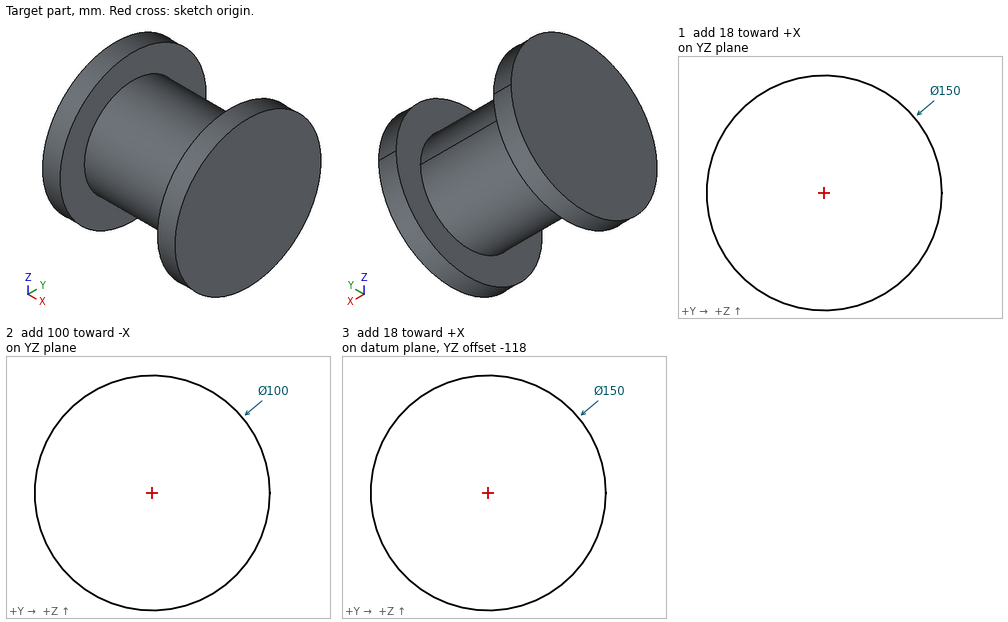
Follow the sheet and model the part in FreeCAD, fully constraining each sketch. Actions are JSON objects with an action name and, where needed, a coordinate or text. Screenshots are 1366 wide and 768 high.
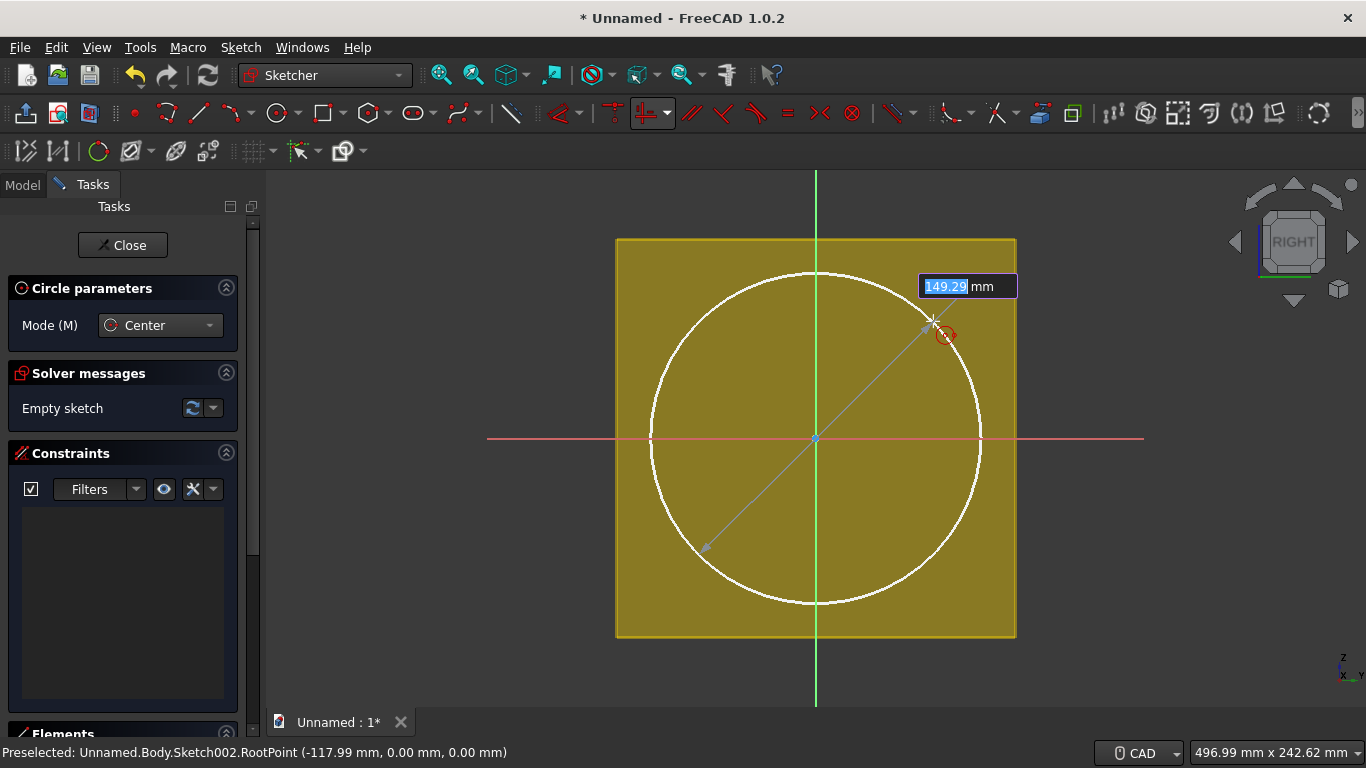
{"action": "type", "text": "150"}
{"action": "key", "text": "Return"}
{"action": "key", "text": "Escape"}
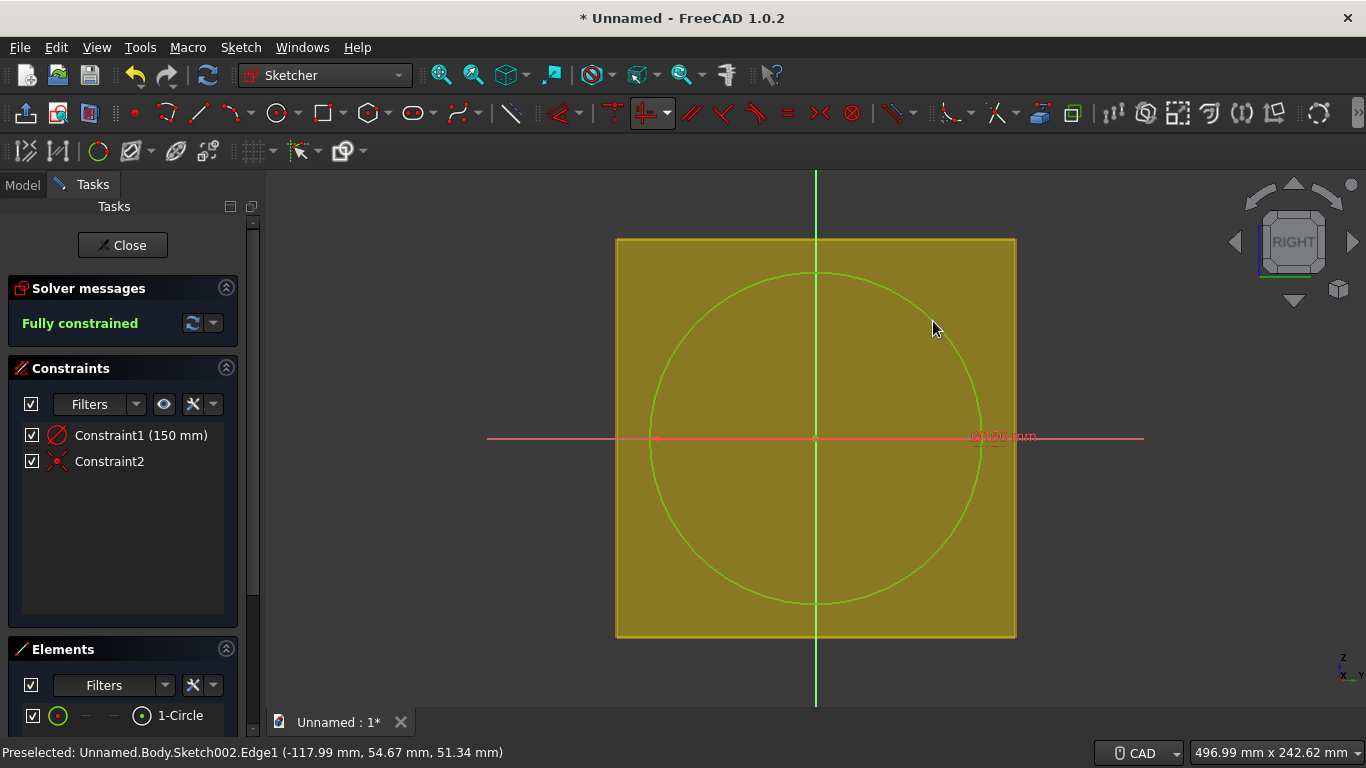
{"action": "left_click", "coordinate": [123, 245]}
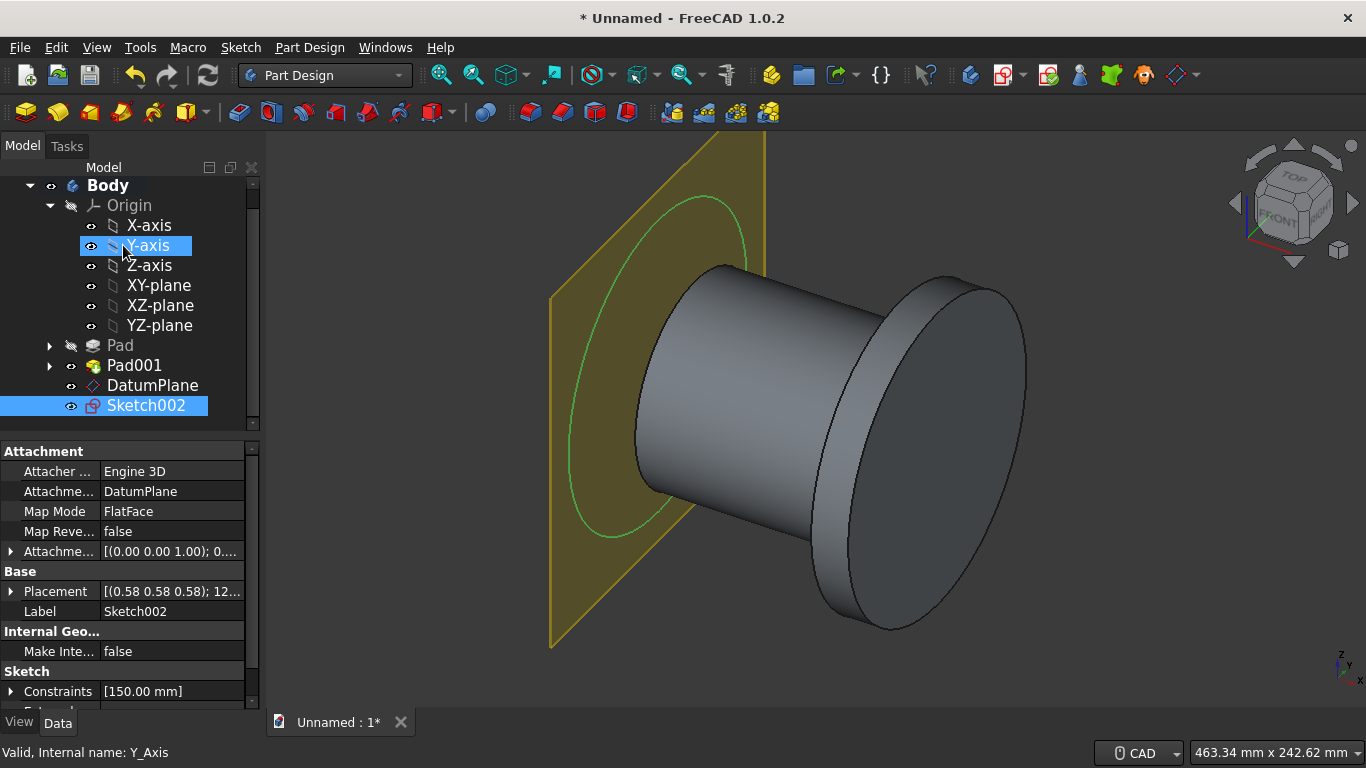
{"action": "left_click", "coordinate": [26, 112]}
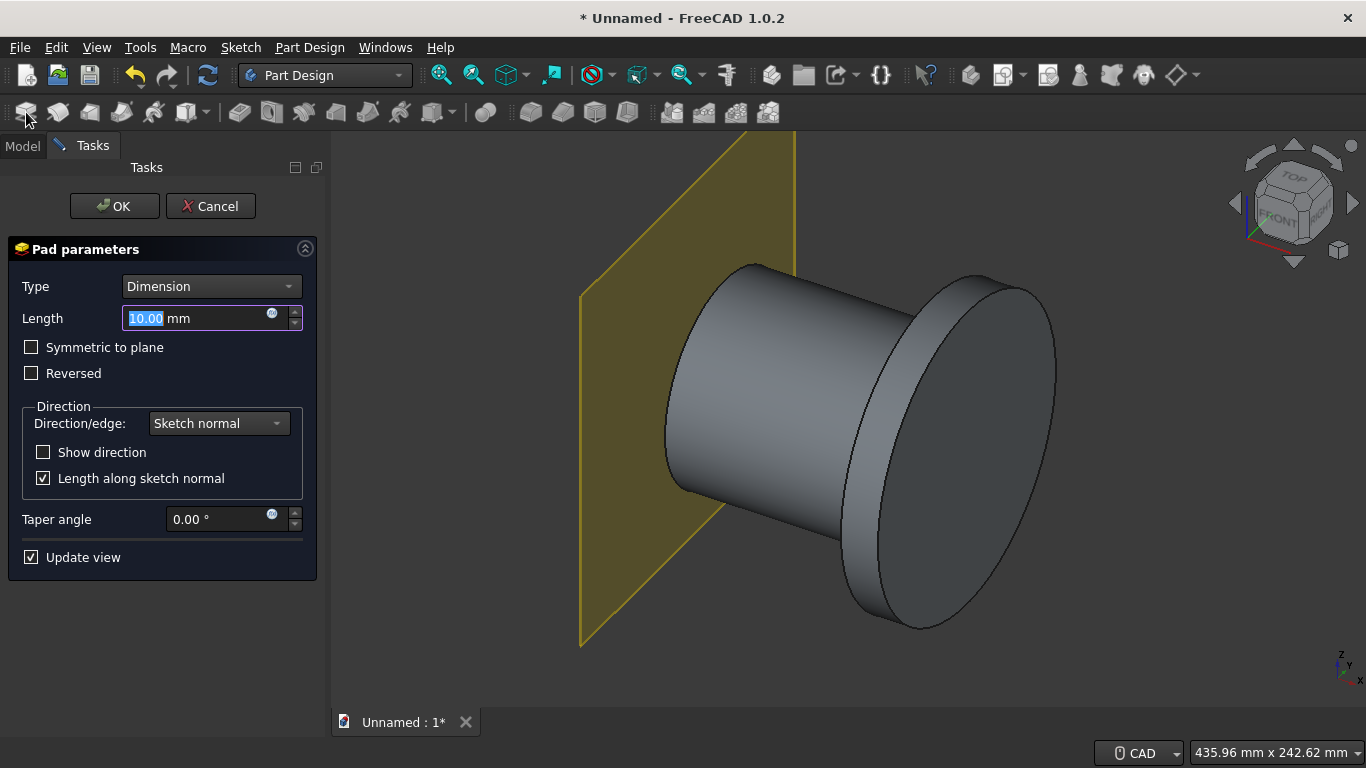
{"action": "type", "text": "18"}
{"action": "key", "text": "Tab"}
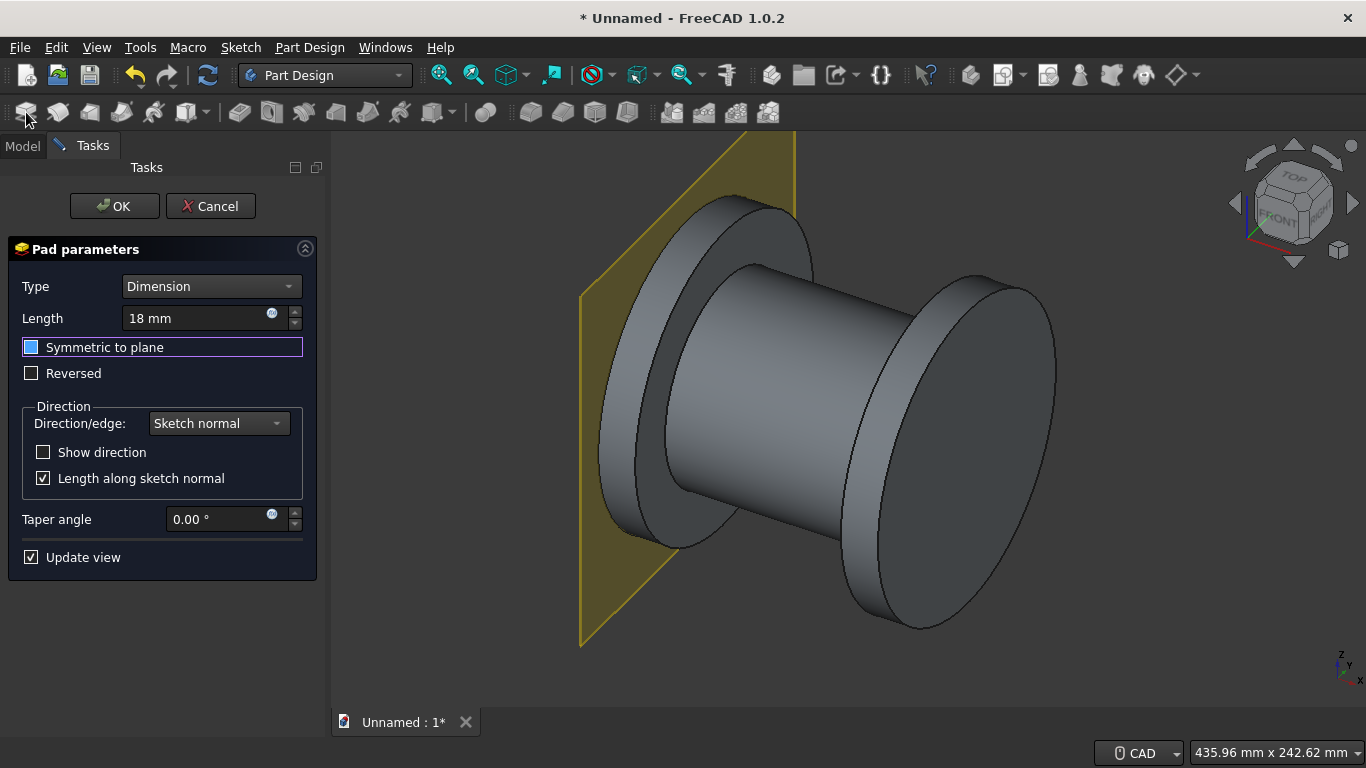
{"action": "left_click", "coordinate": [115, 206]}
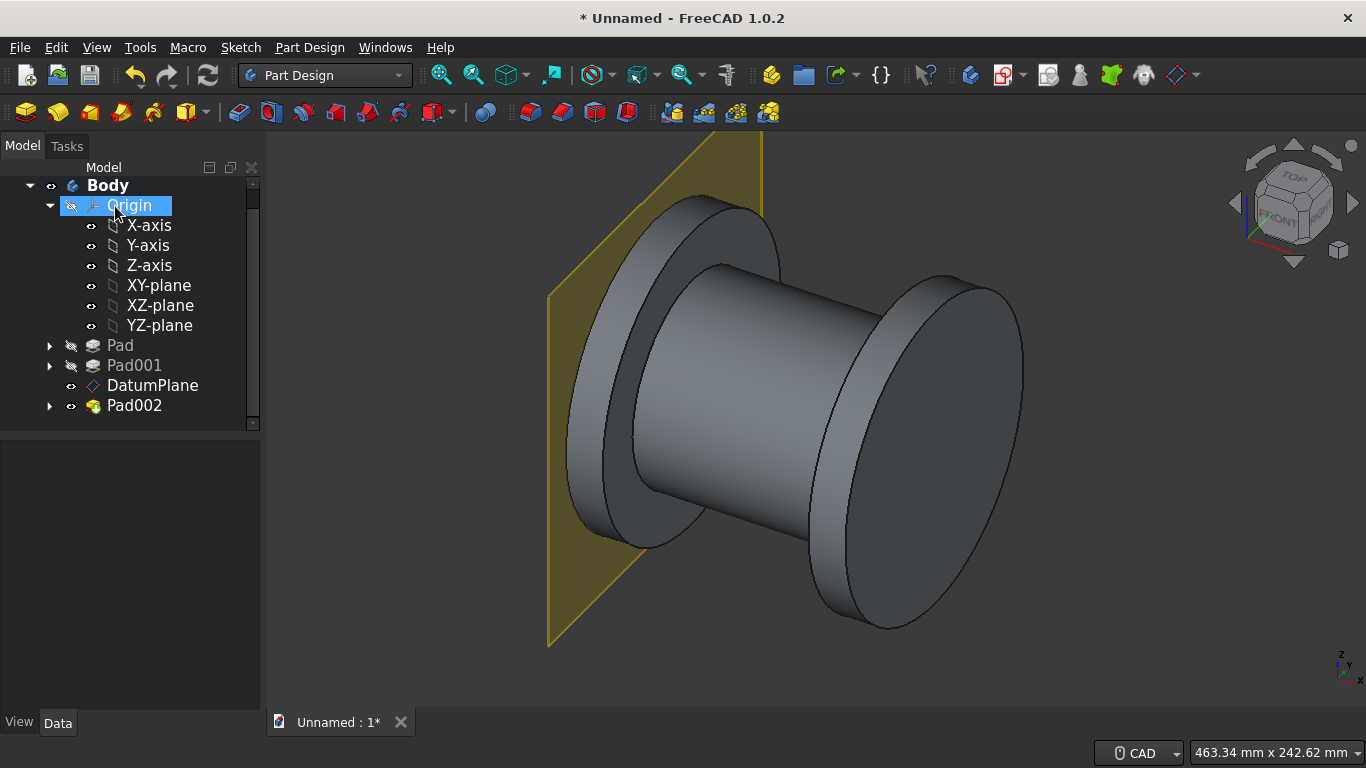
{"action": "left_click", "coordinate": [116, 386]}
{"action": "key", "text": "space"}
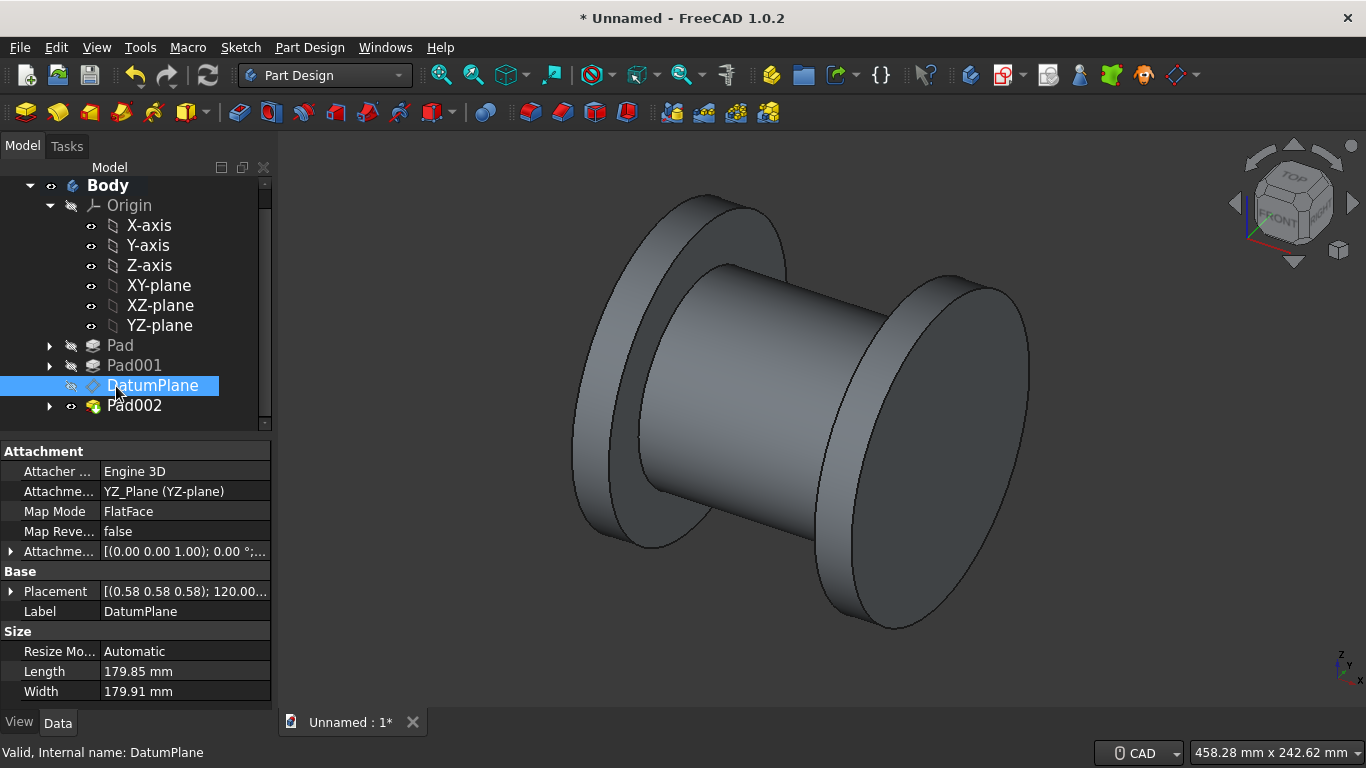
{"action": "key", "text": "0"}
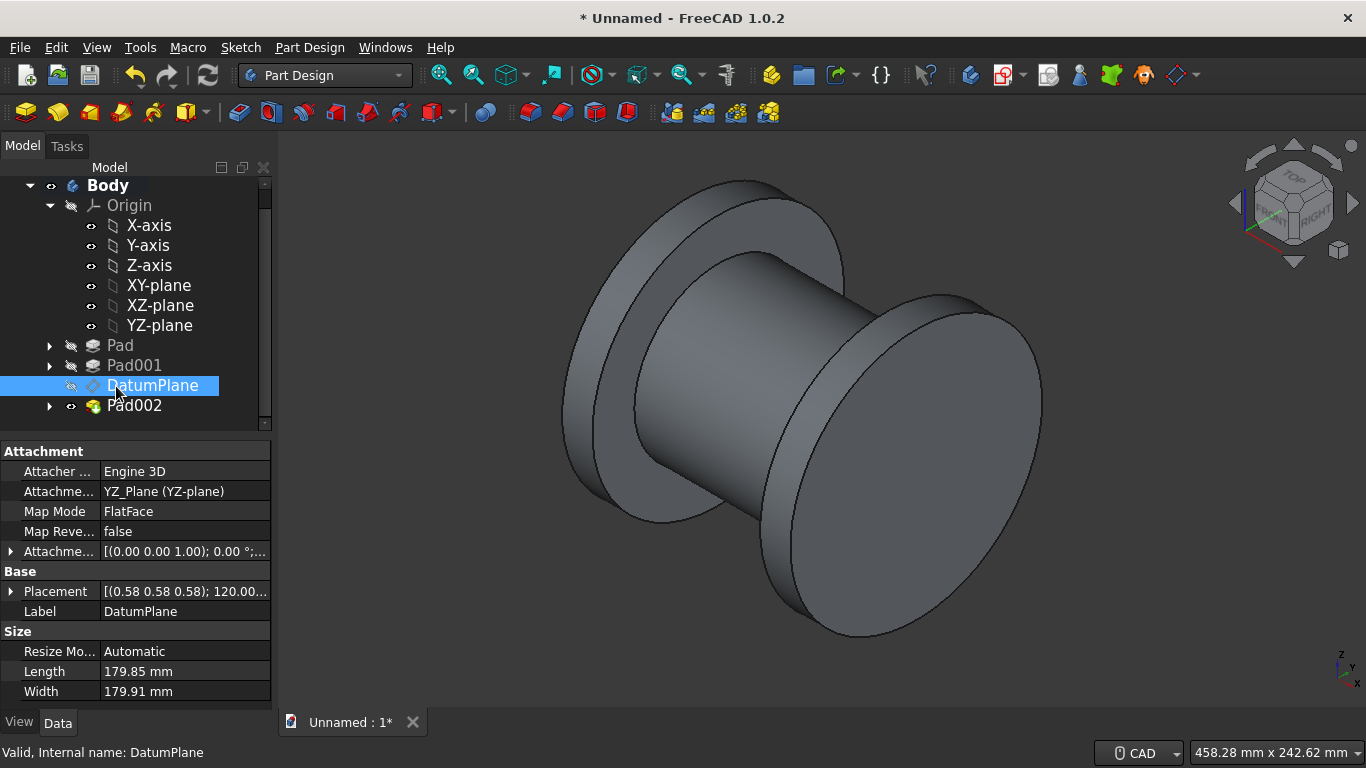
{"action": "left_click", "coordinate": [442, 76]}